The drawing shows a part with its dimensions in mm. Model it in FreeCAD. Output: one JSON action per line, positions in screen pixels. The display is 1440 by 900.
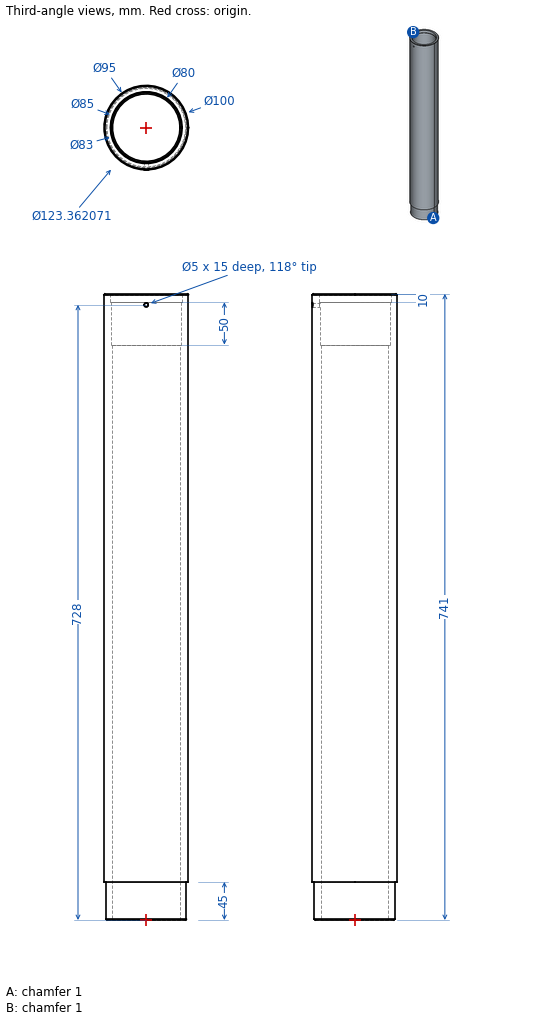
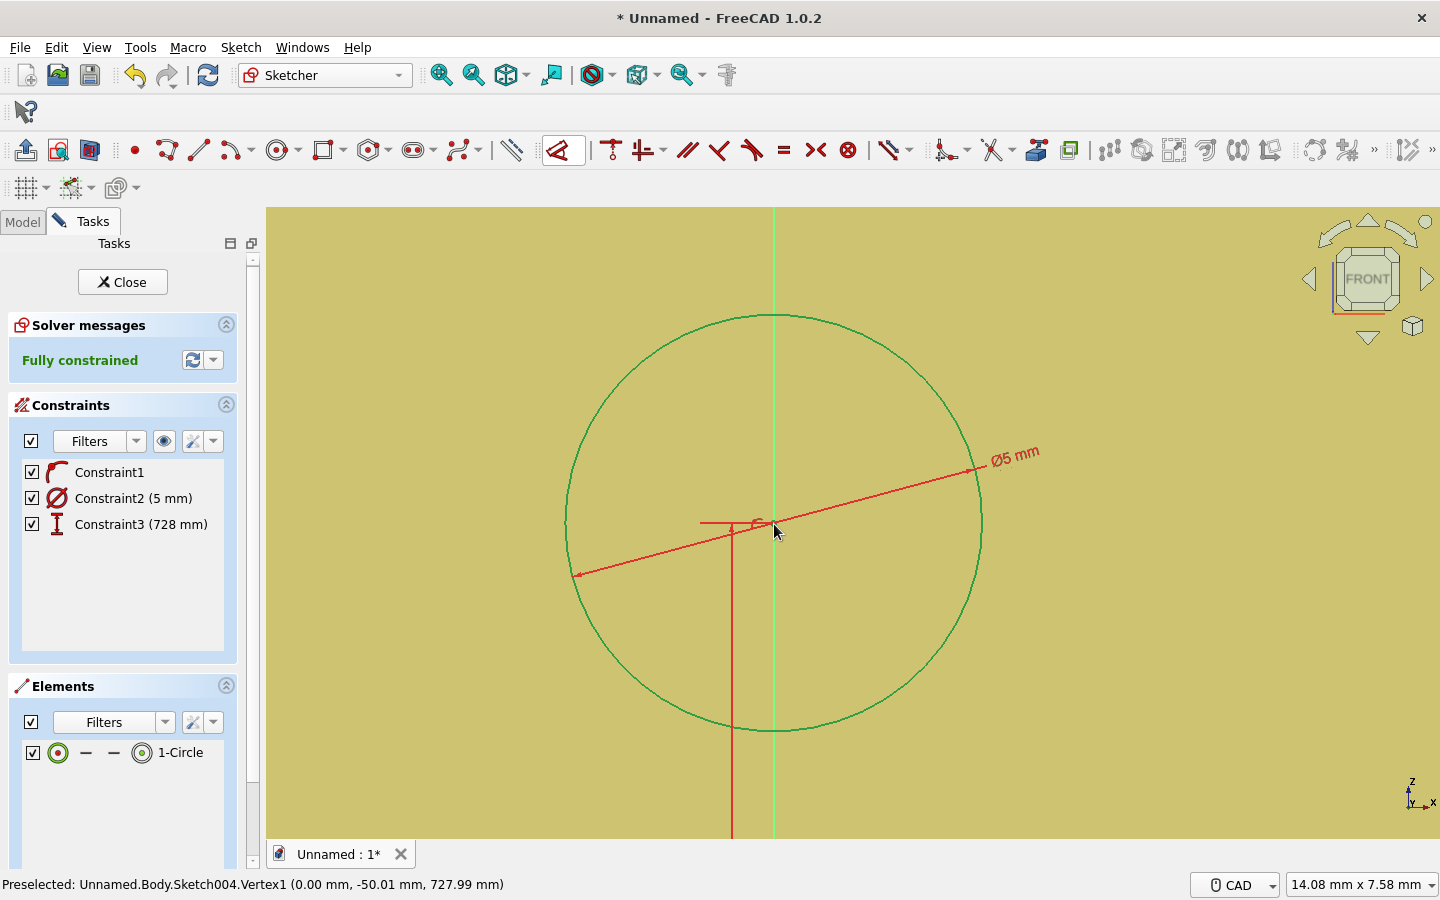
{"action": "left_click", "coordinate": [123, 282]}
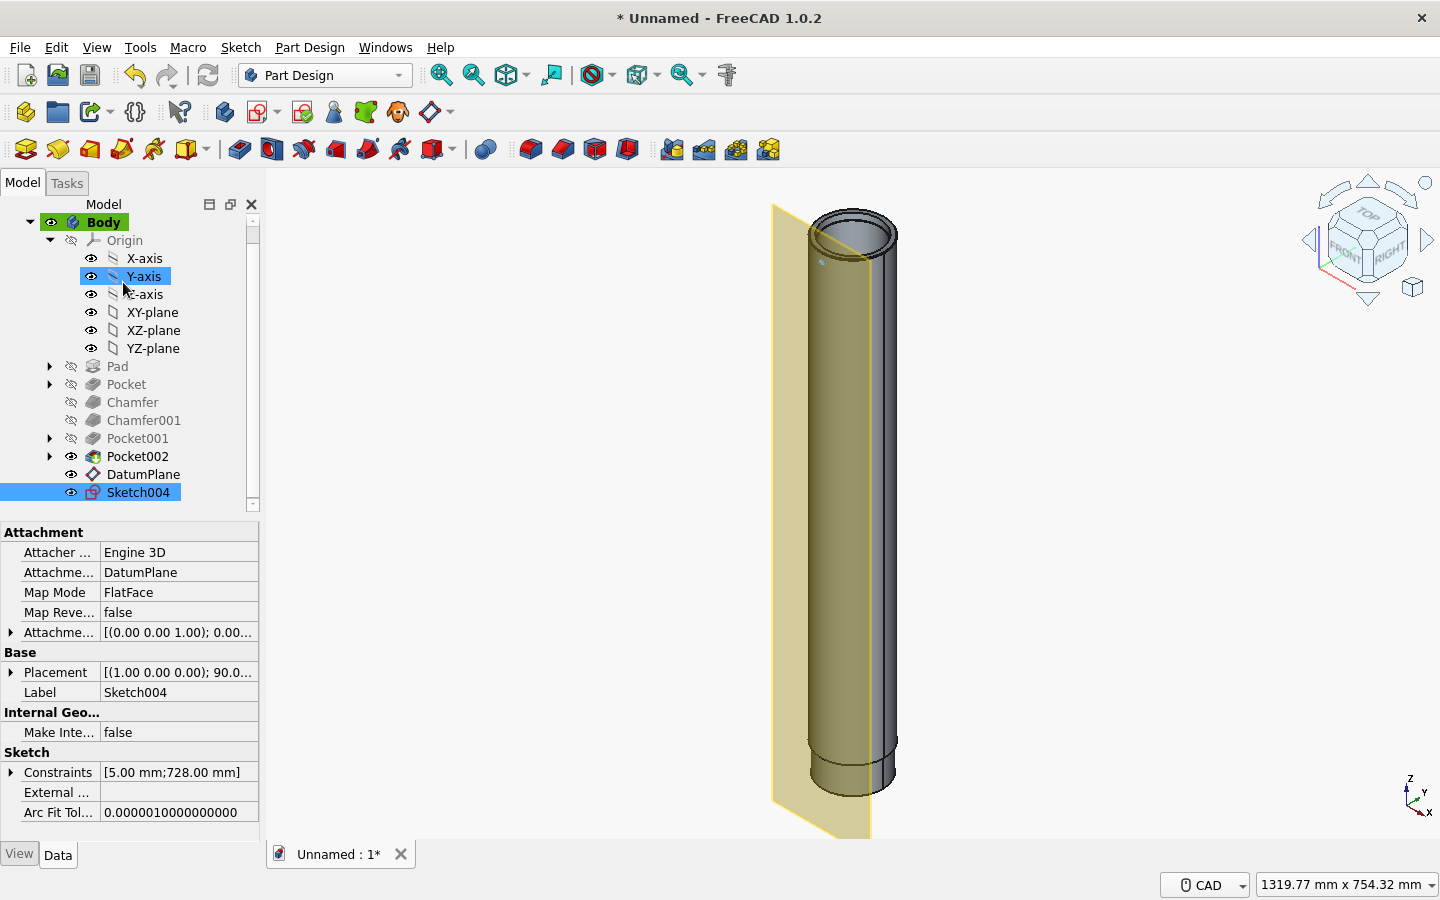
{"action": "left_click", "coordinate": [272, 150]}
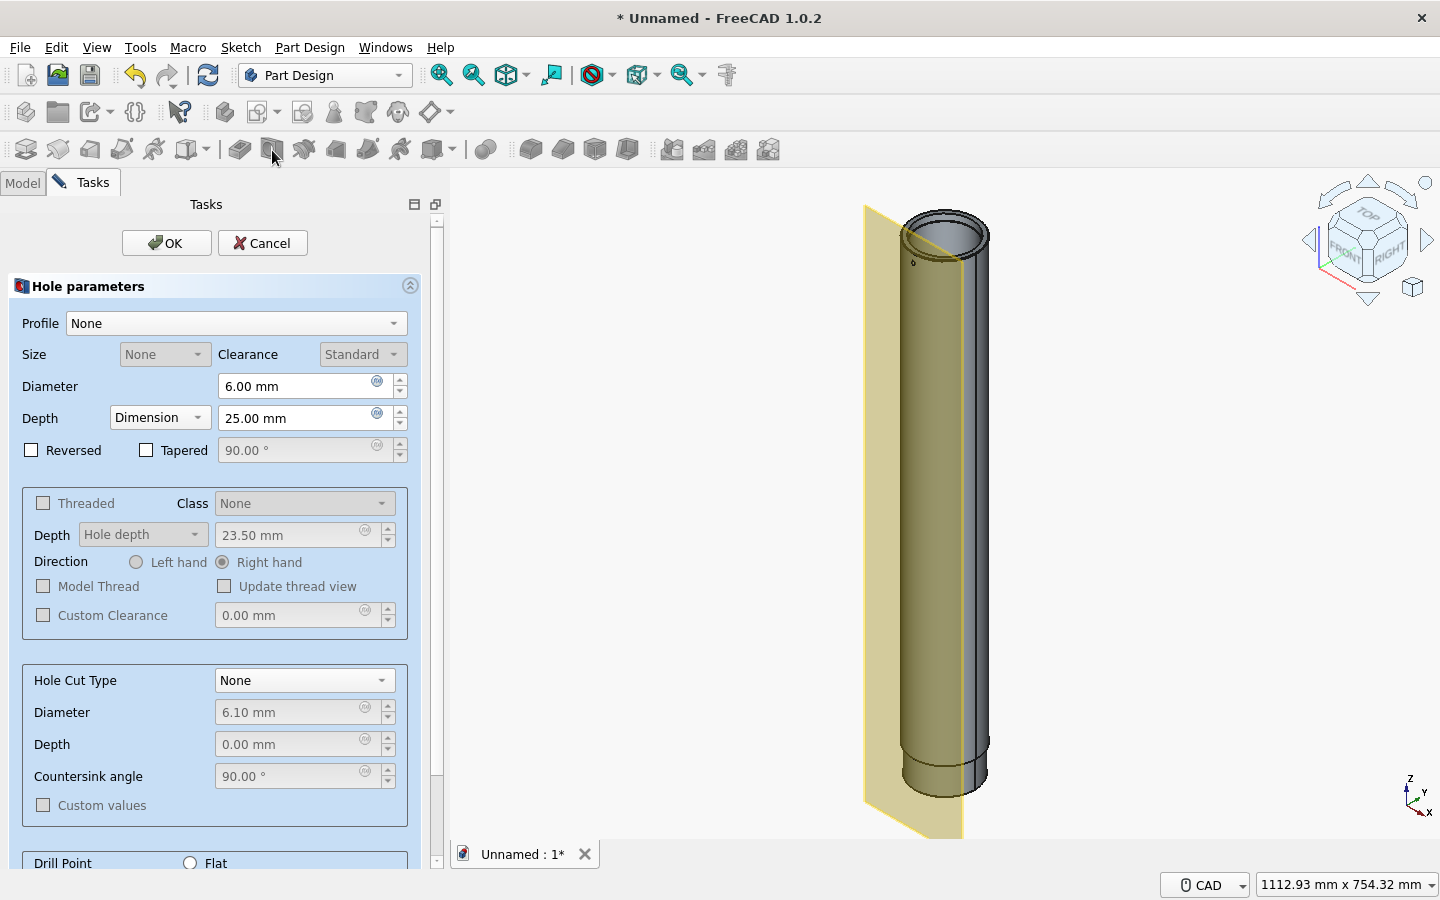
{"action": "triple_click", "coordinate": [305, 386]}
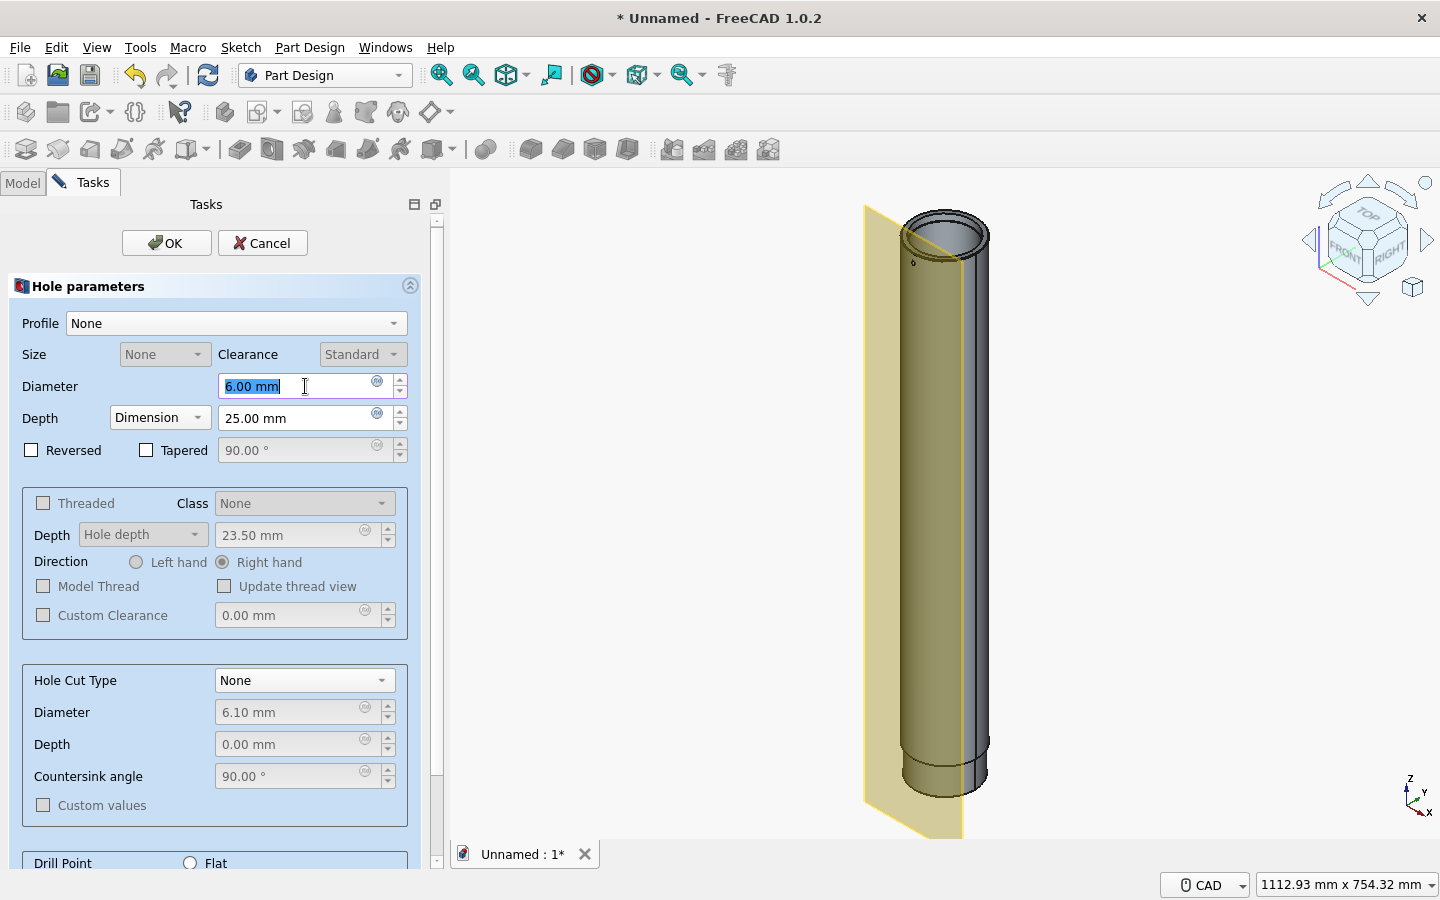
{"action": "type", "text": "5"}
{"action": "key", "text": "Tab"}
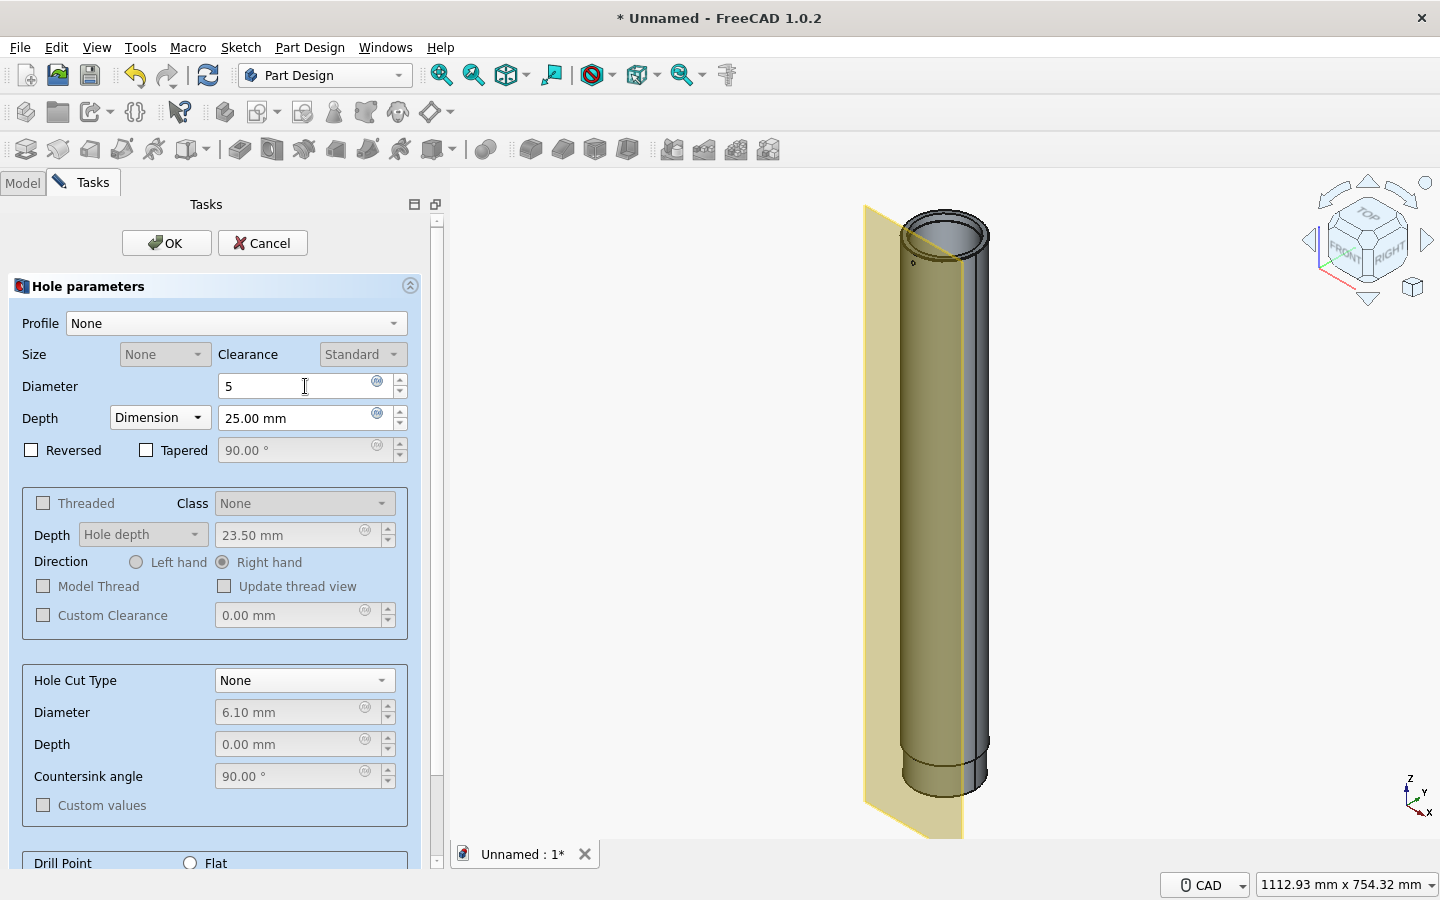
{"action": "triple_click", "coordinate": [305, 418]}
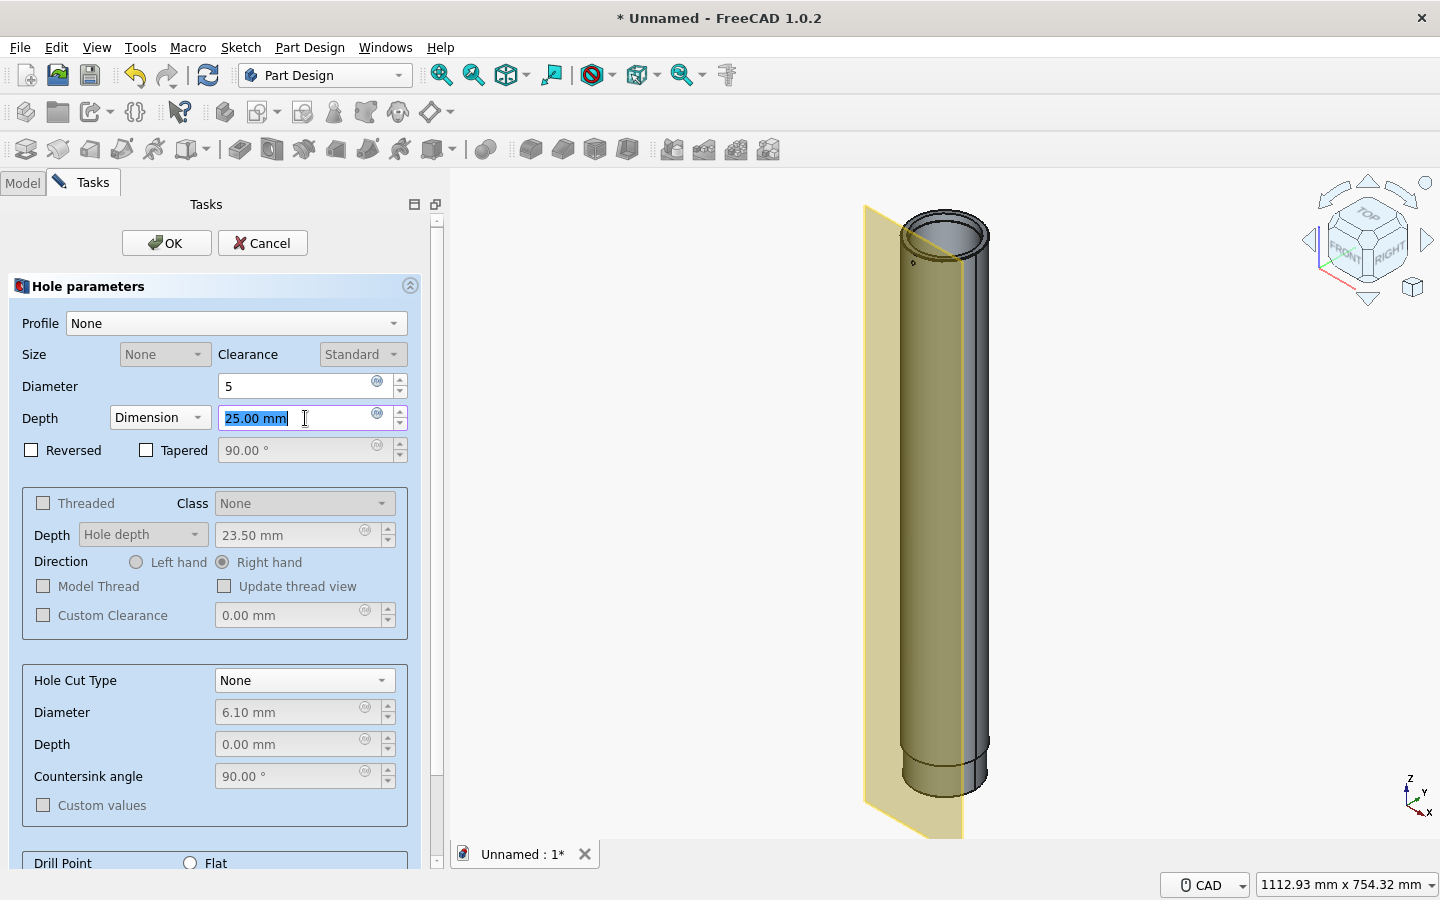
{"action": "type", "text": "15"}
{"action": "key", "text": "Tab"}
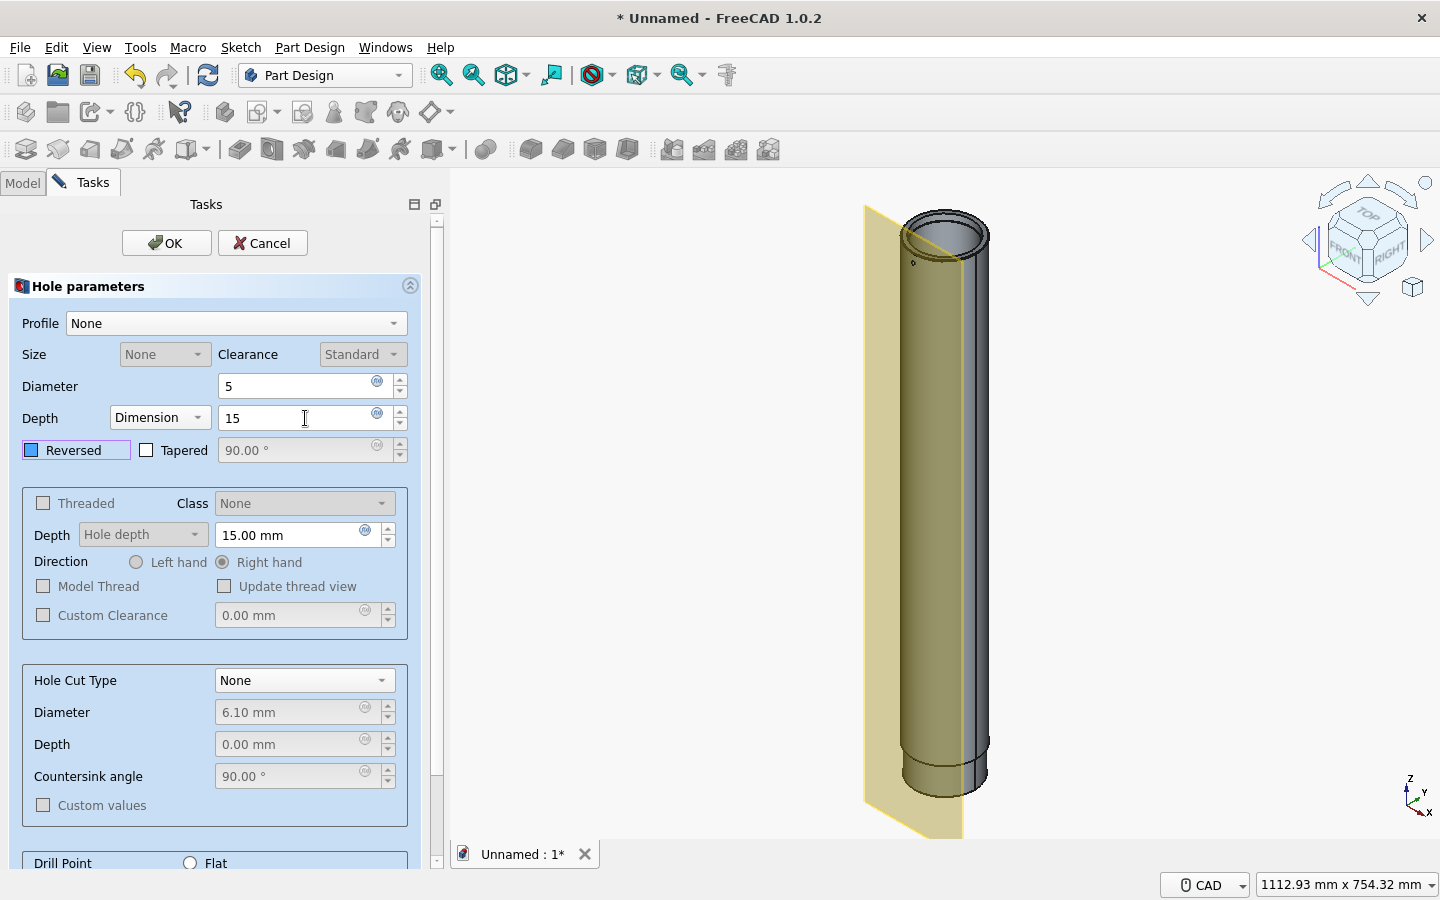
{"action": "left_click", "coordinate": [167, 243]}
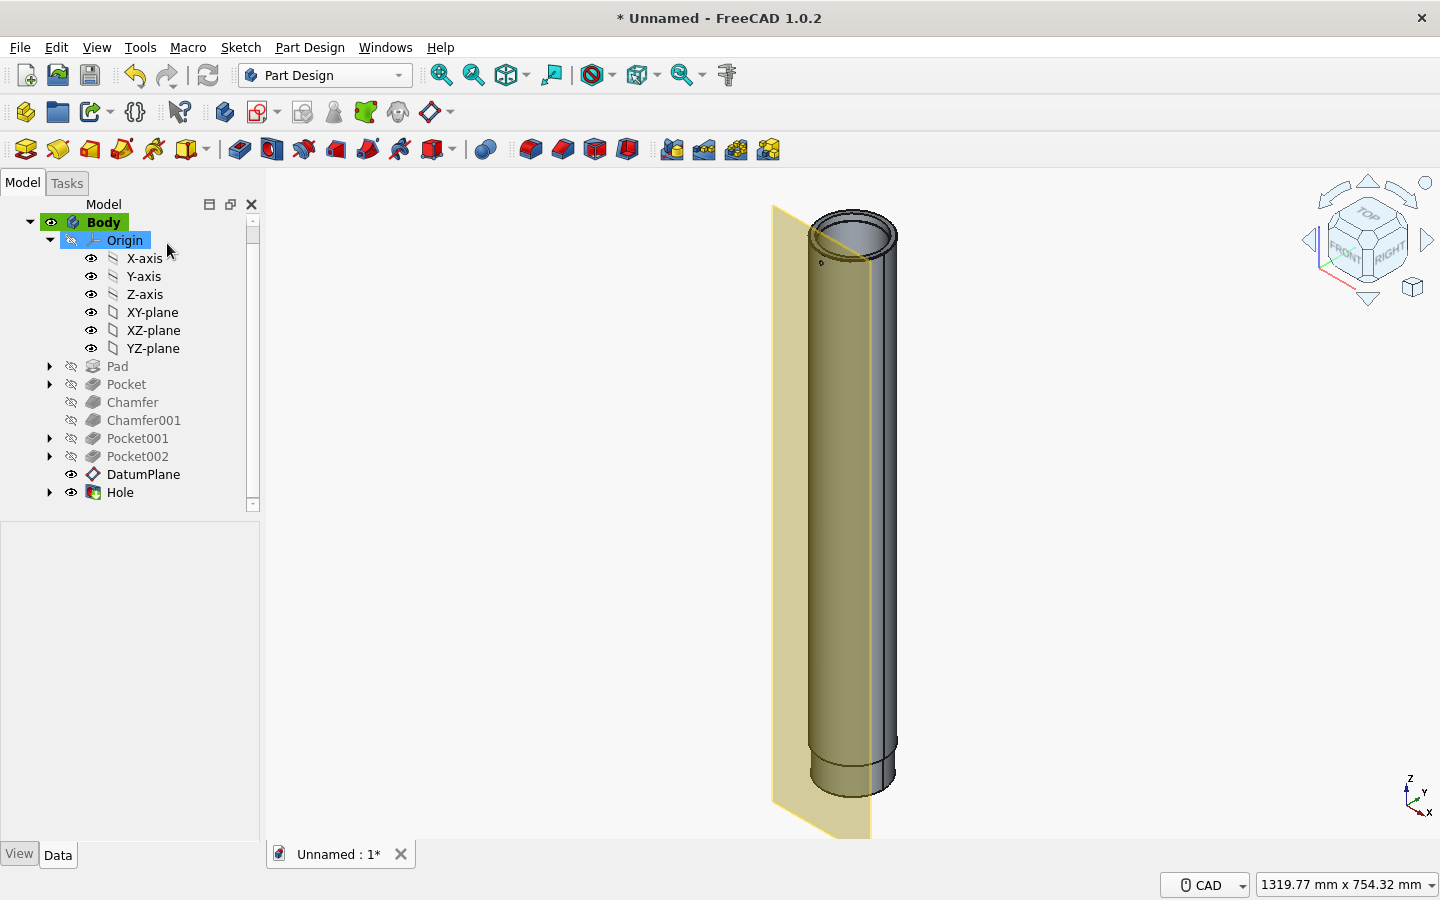
{"action": "left_click", "coordinate": [116, 474]}
{"action": "key", "text": "space"}